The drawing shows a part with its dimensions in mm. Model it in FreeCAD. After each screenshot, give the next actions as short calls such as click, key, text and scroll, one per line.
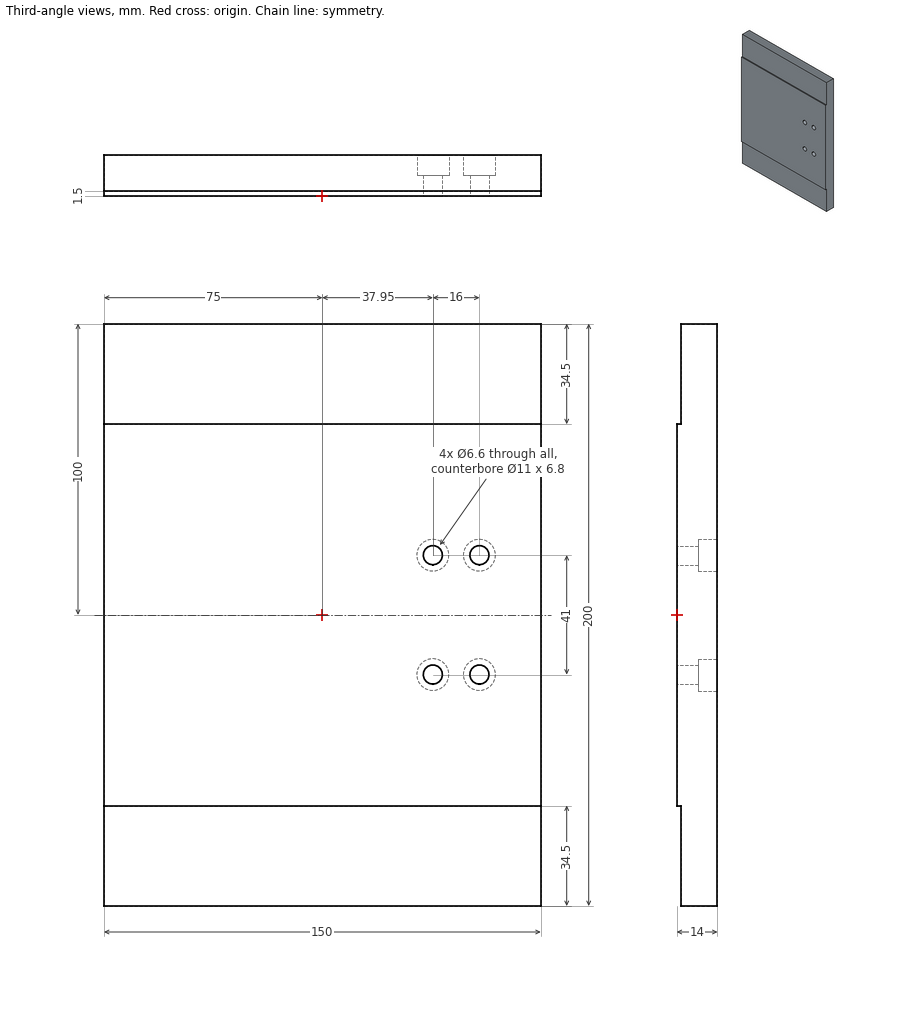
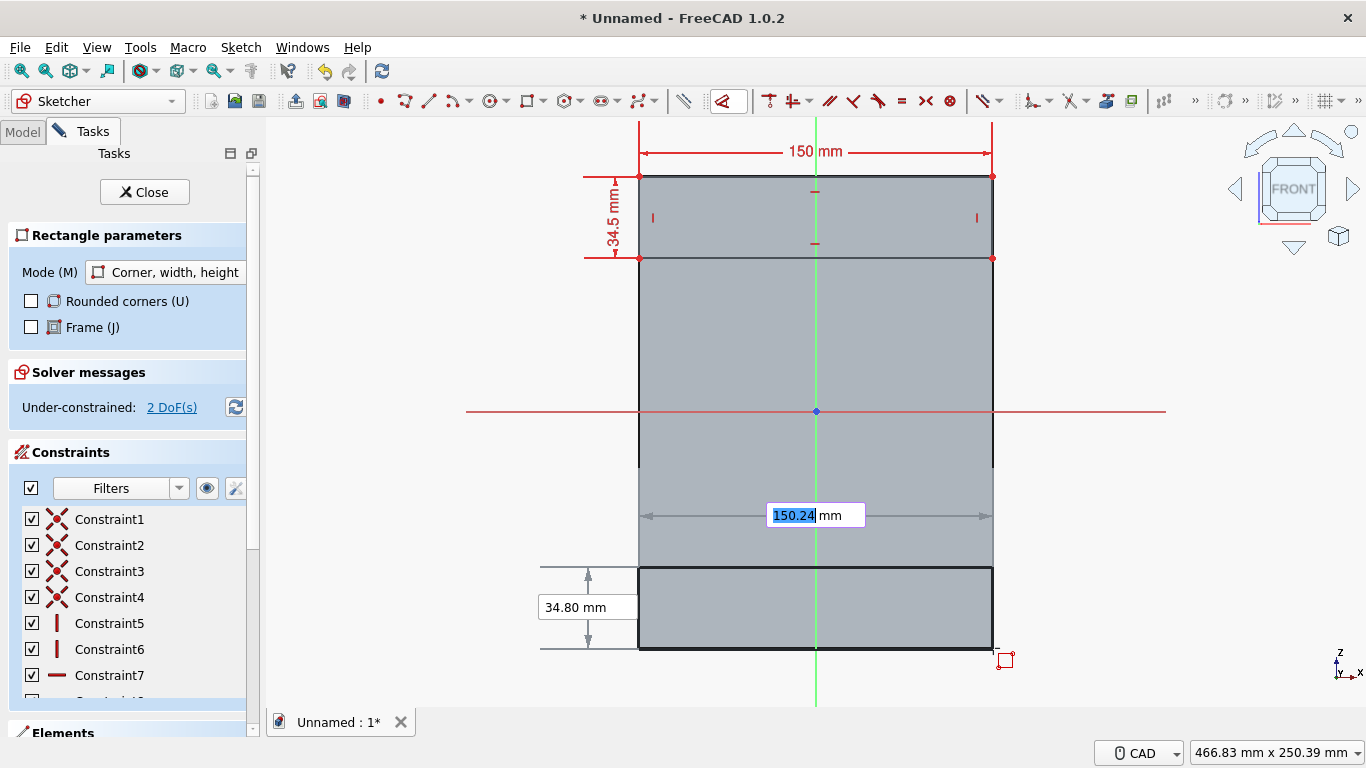
text(150)
key(Tab)
text(34.5)
key(Return)
key(Escape)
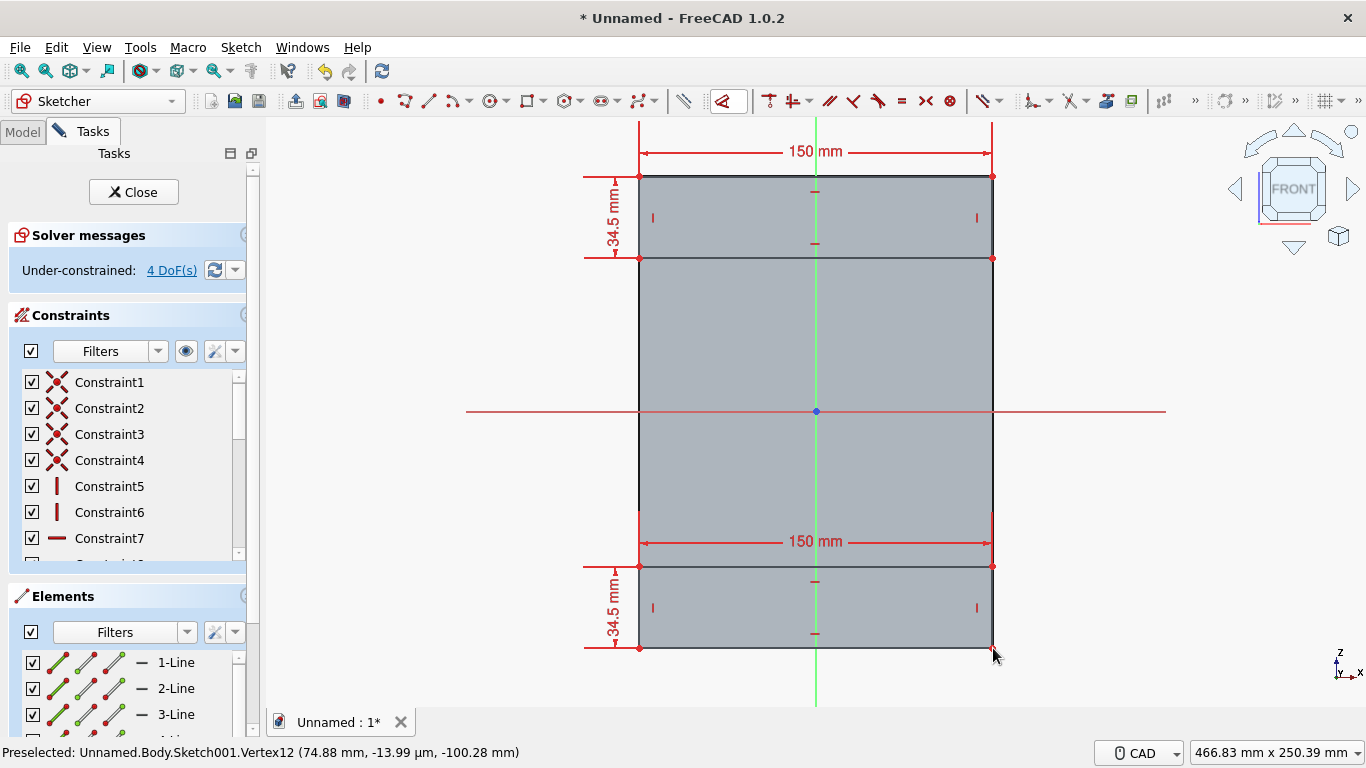
click(639, 258)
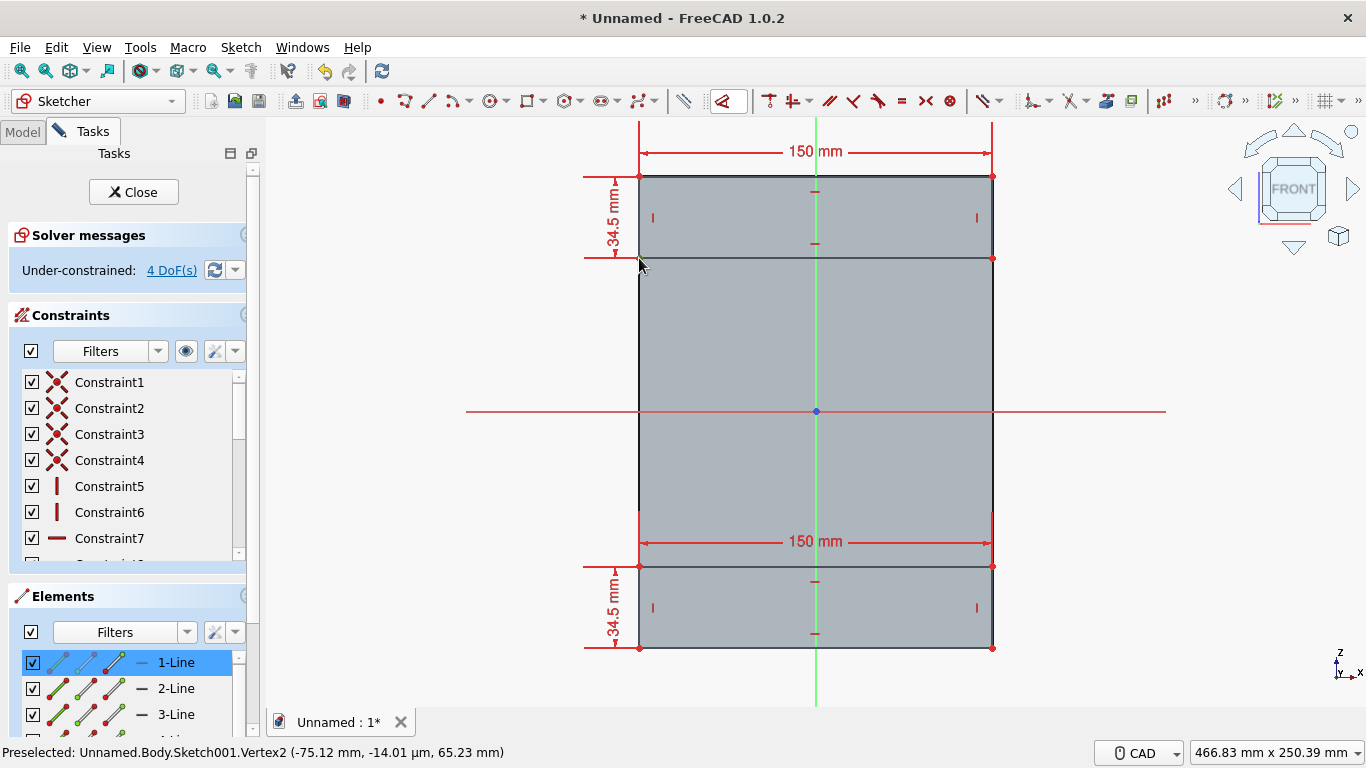
click(639, 567)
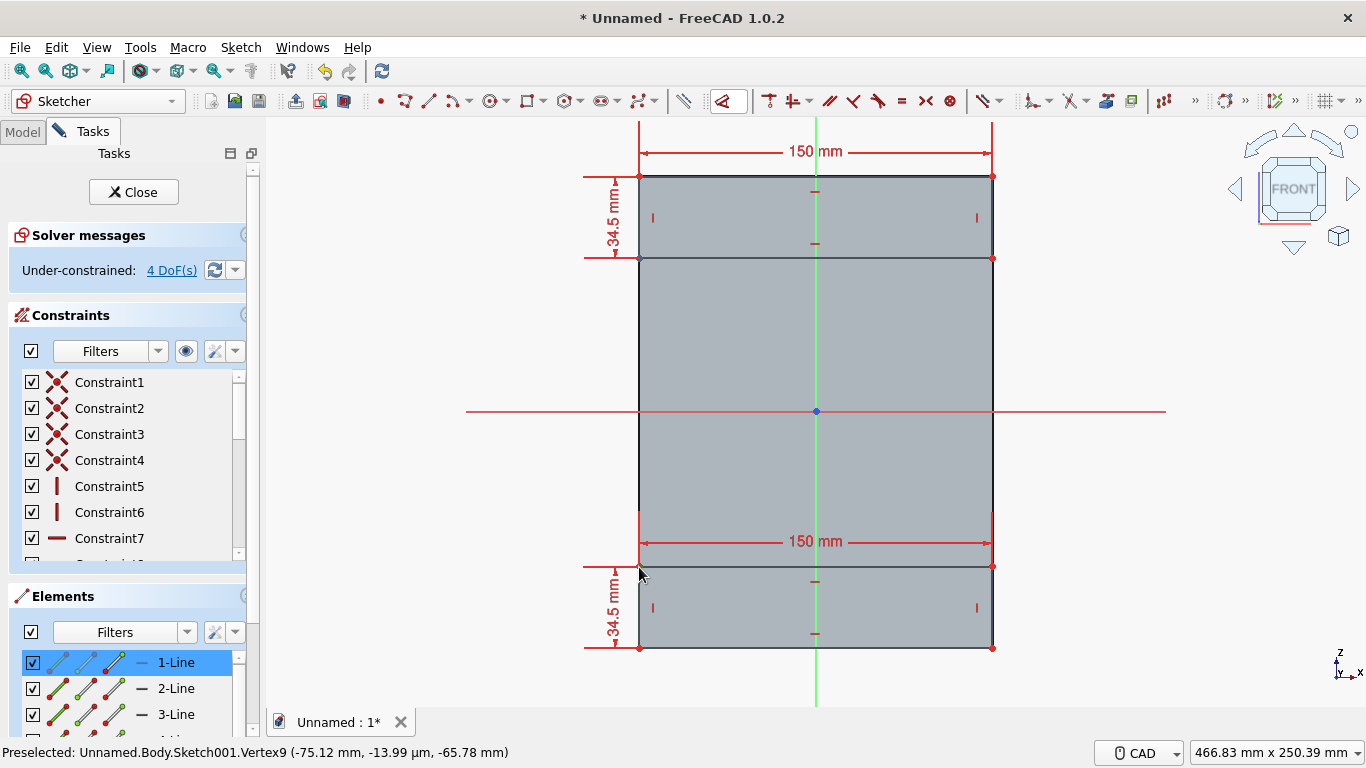
click(488, 412)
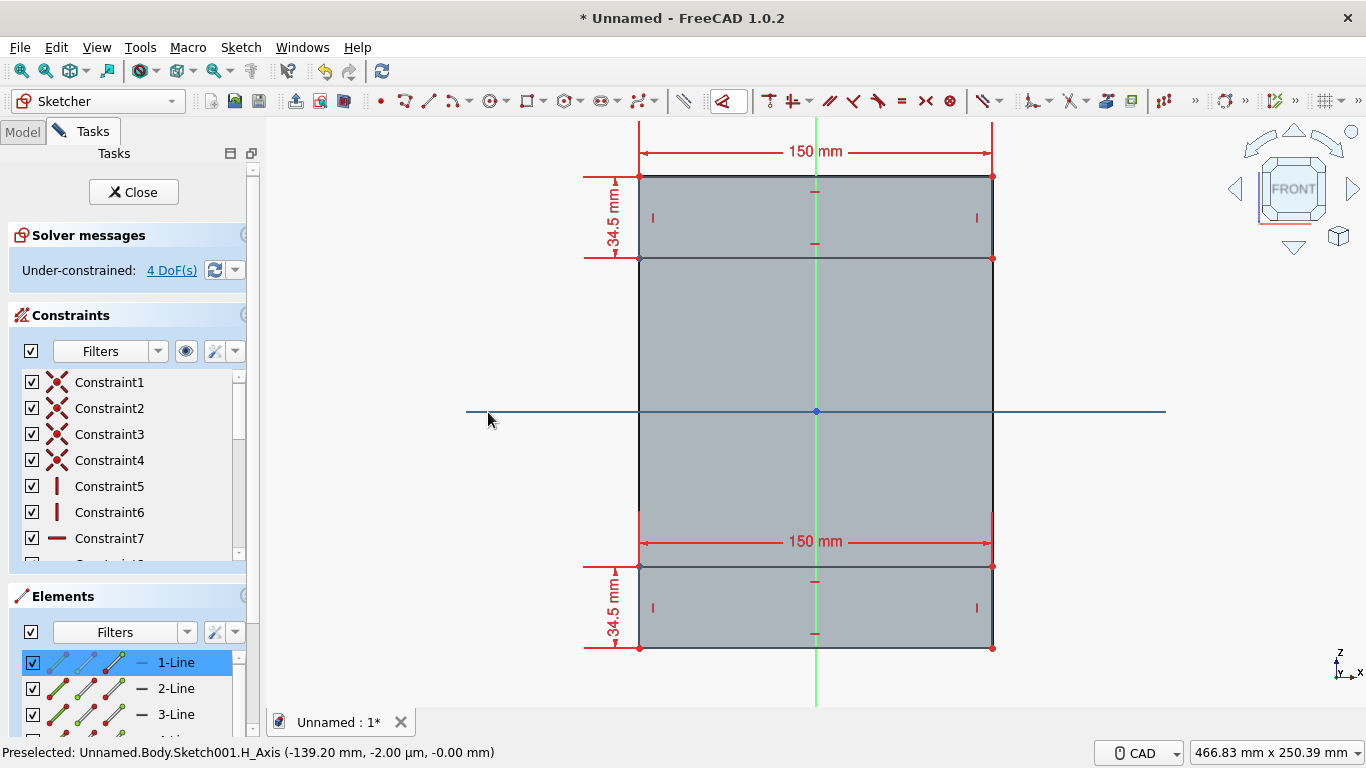
key(s)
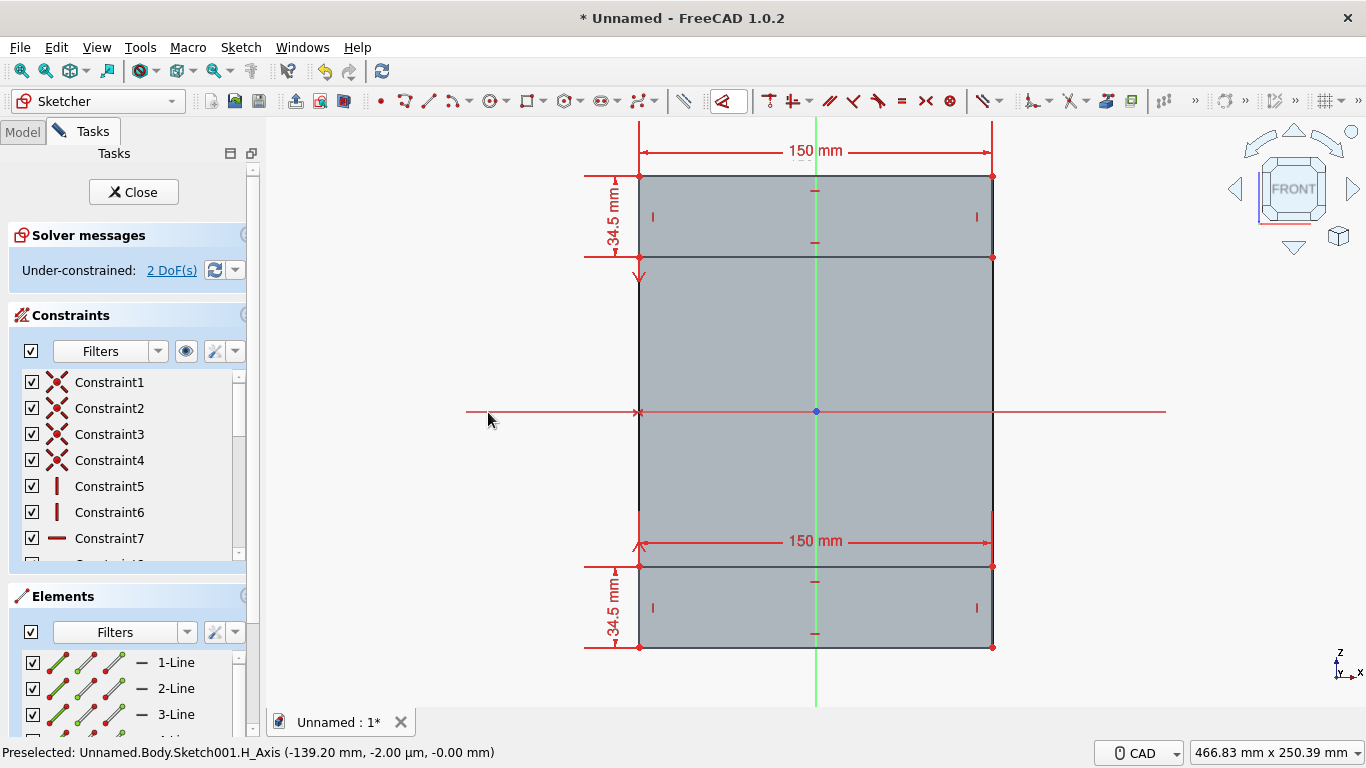
key(d)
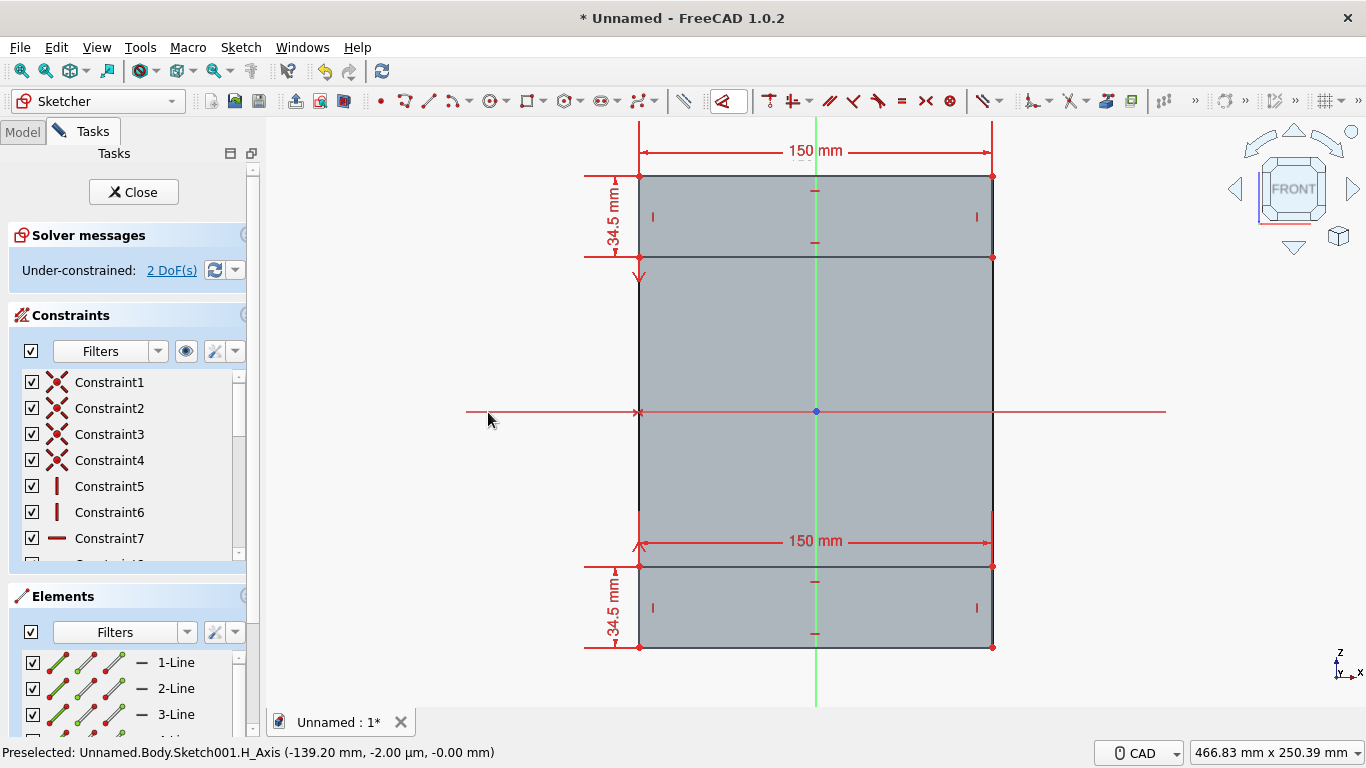
click(639, 176)
click(727, 446)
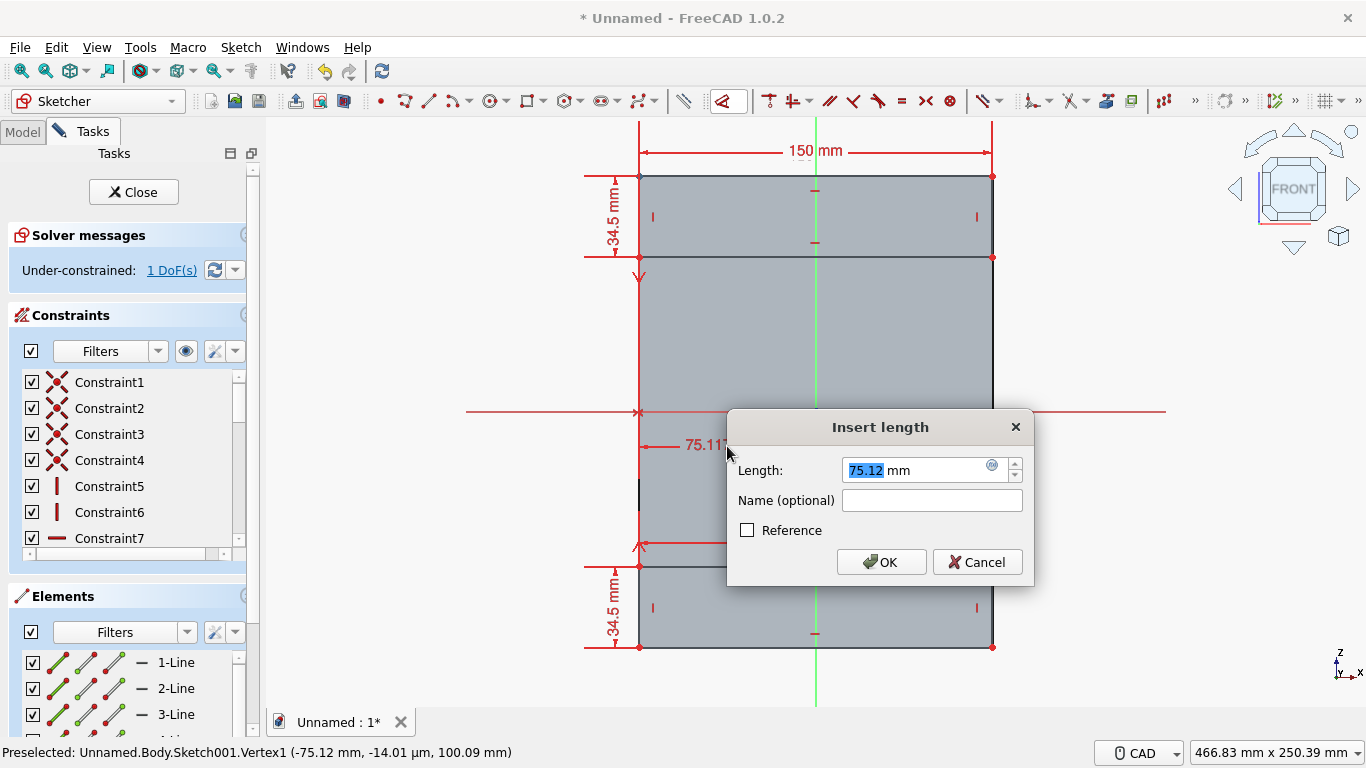
text(75)
key(Return)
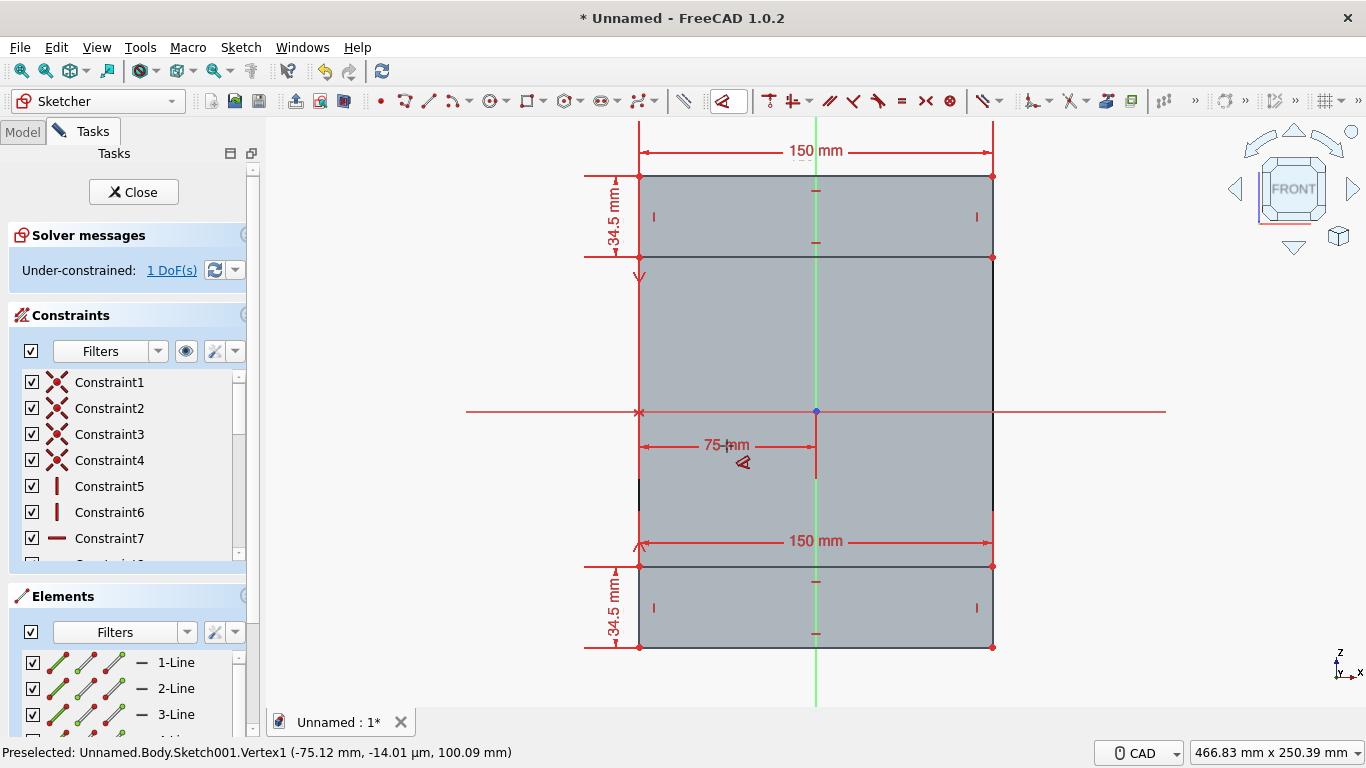
click(639, 176)
click(605, 294)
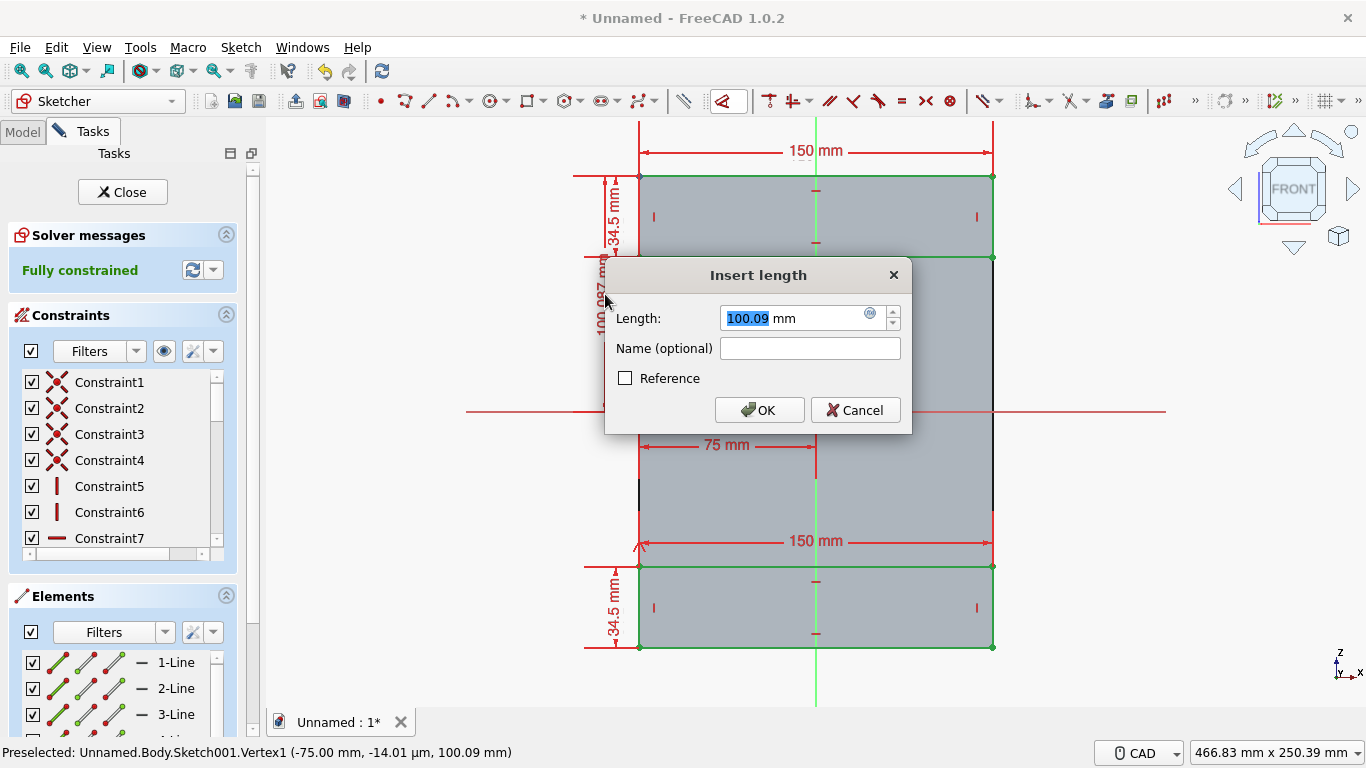
text(100)
key(Return)
key(Escape)